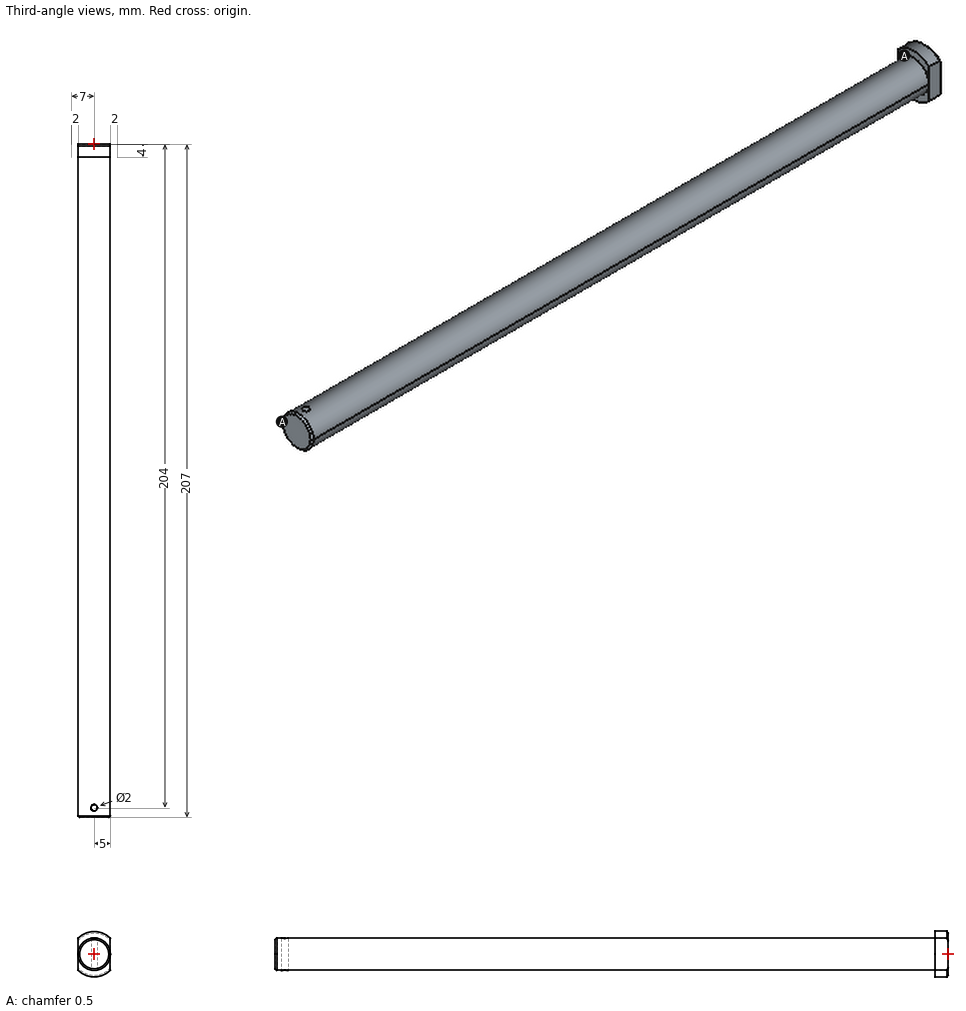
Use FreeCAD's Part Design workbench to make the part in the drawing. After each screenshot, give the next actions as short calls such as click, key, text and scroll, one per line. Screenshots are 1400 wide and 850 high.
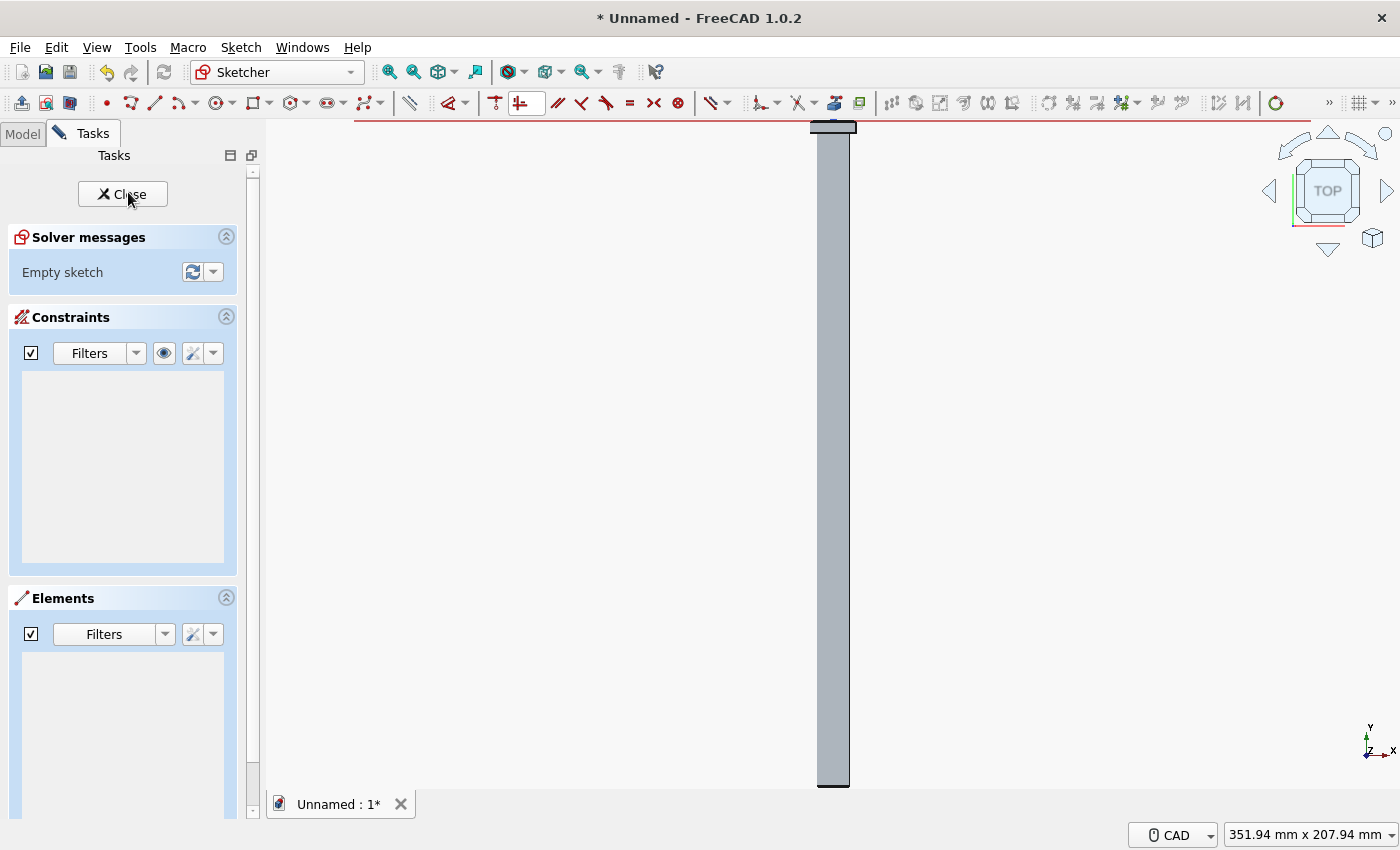
click(70, 104)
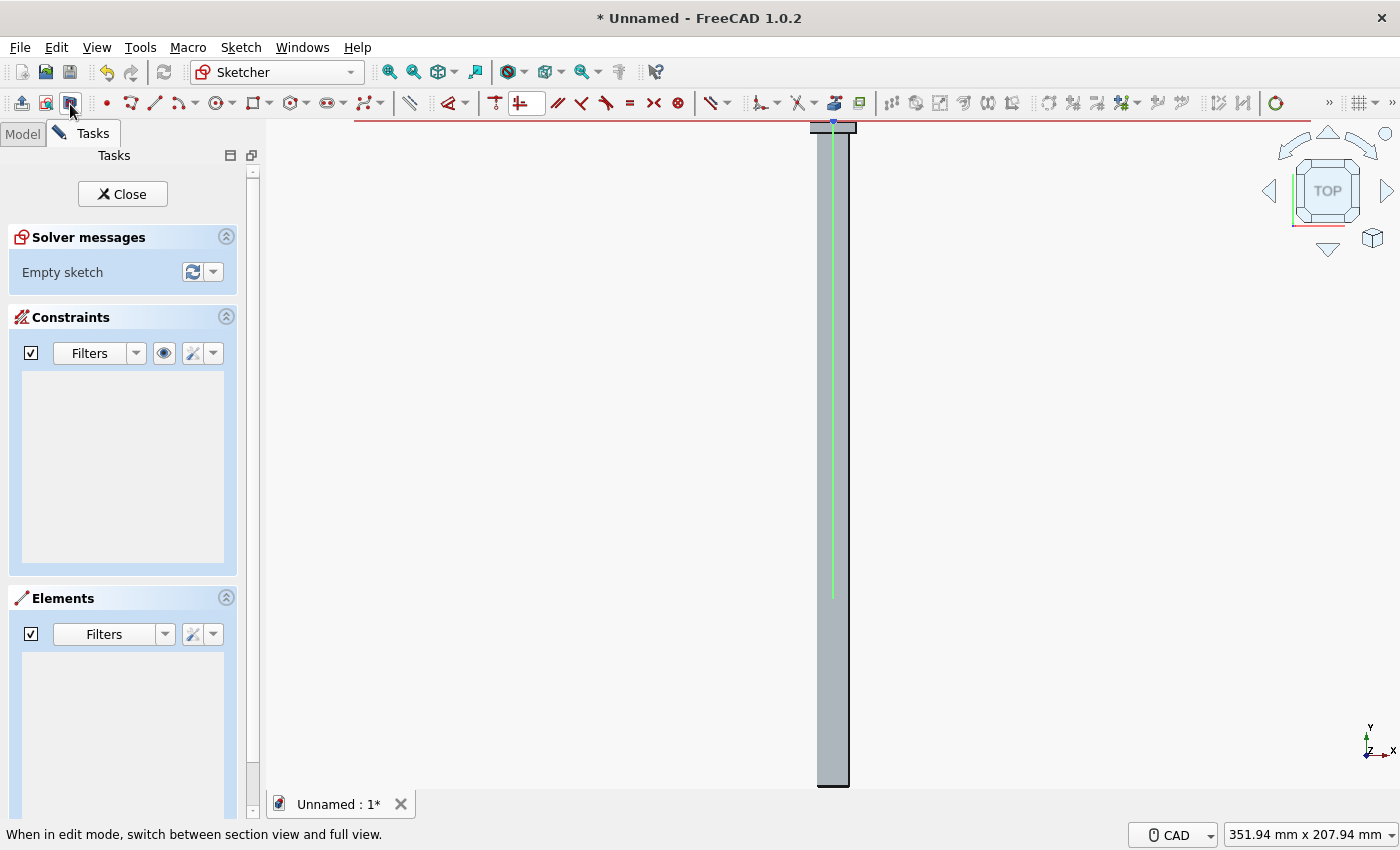
scroll(764, 454, down, 5)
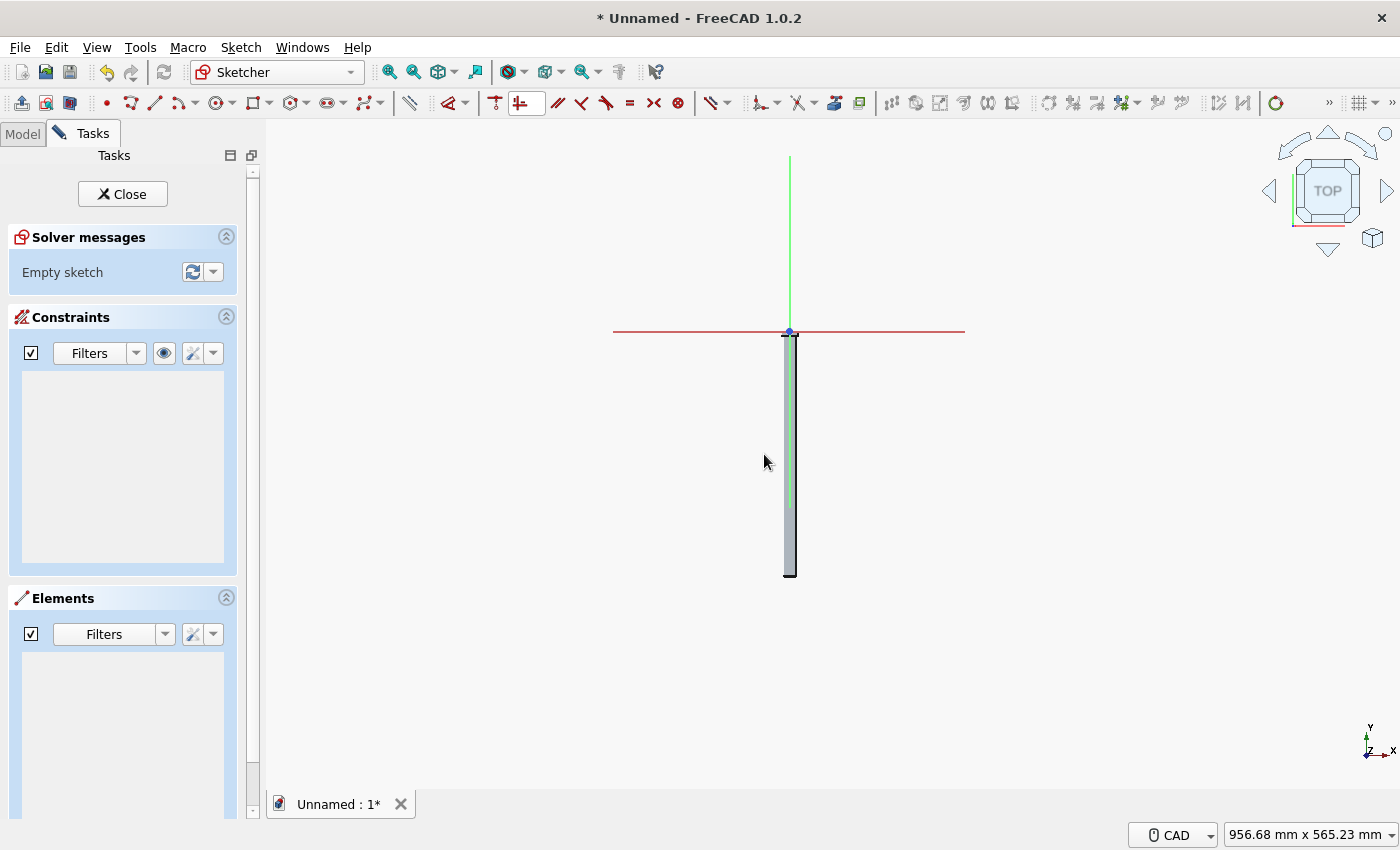
scroll(791, 580, up, 15)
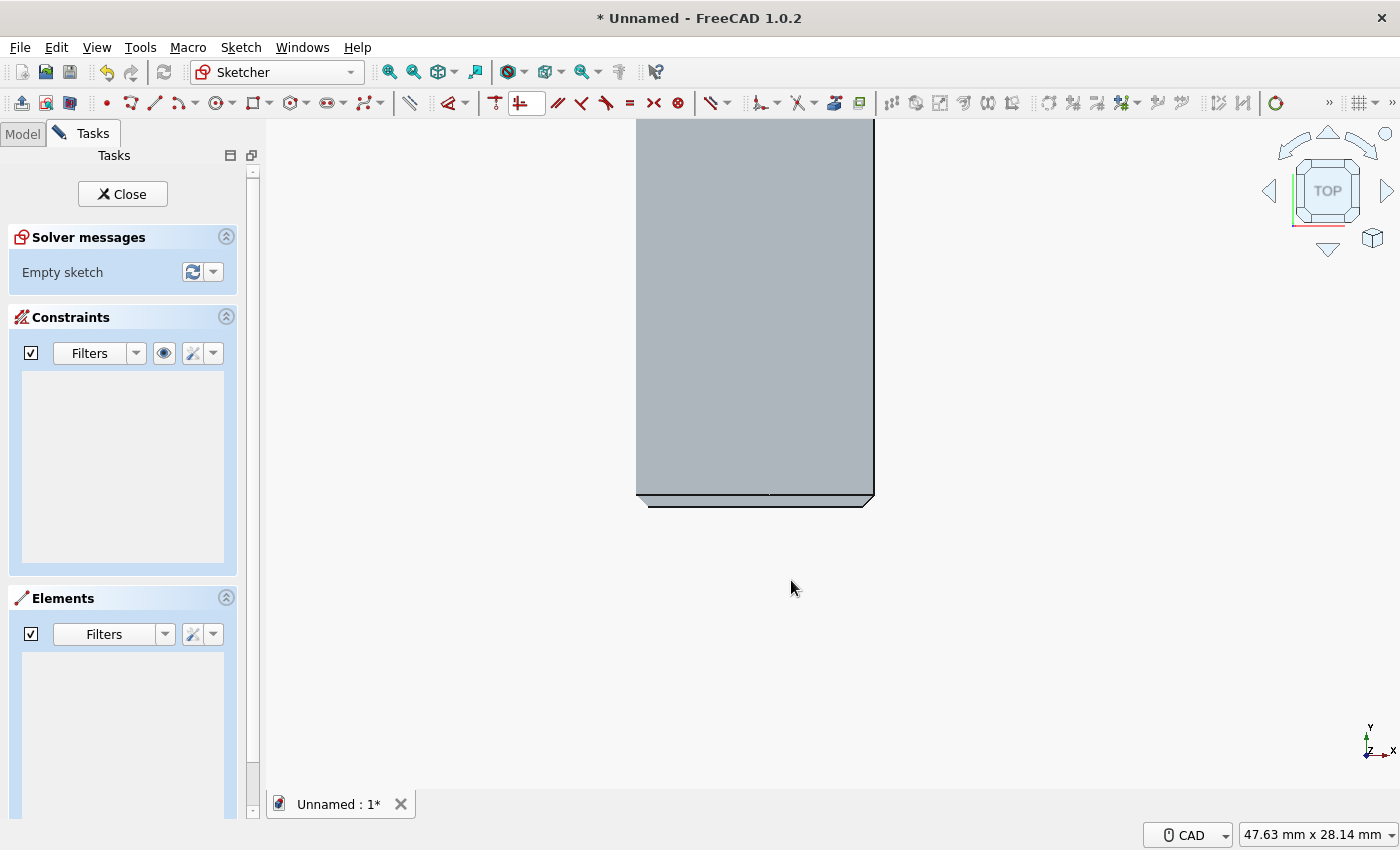
scroll(754, 433, up, 11)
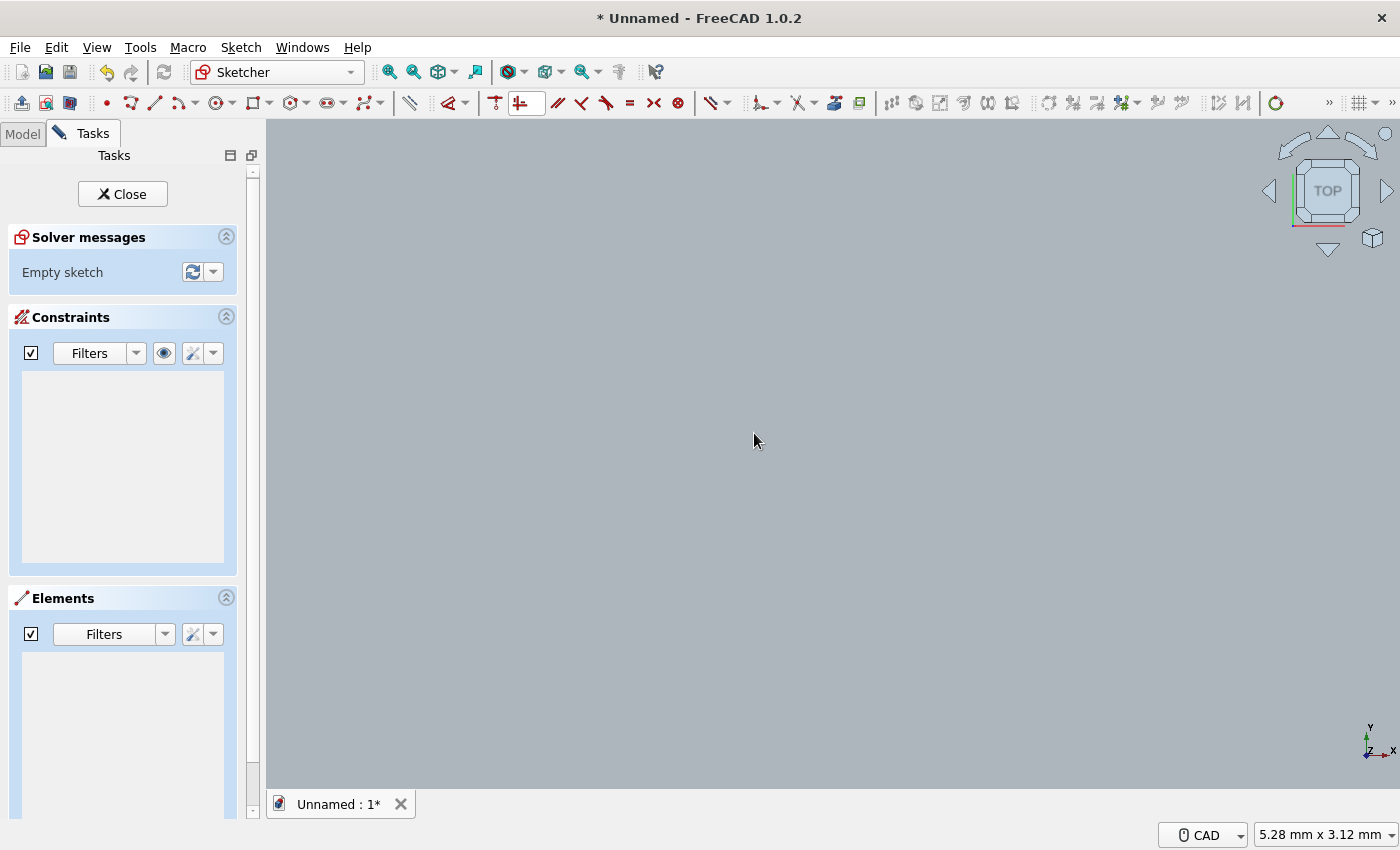
click(216, 104)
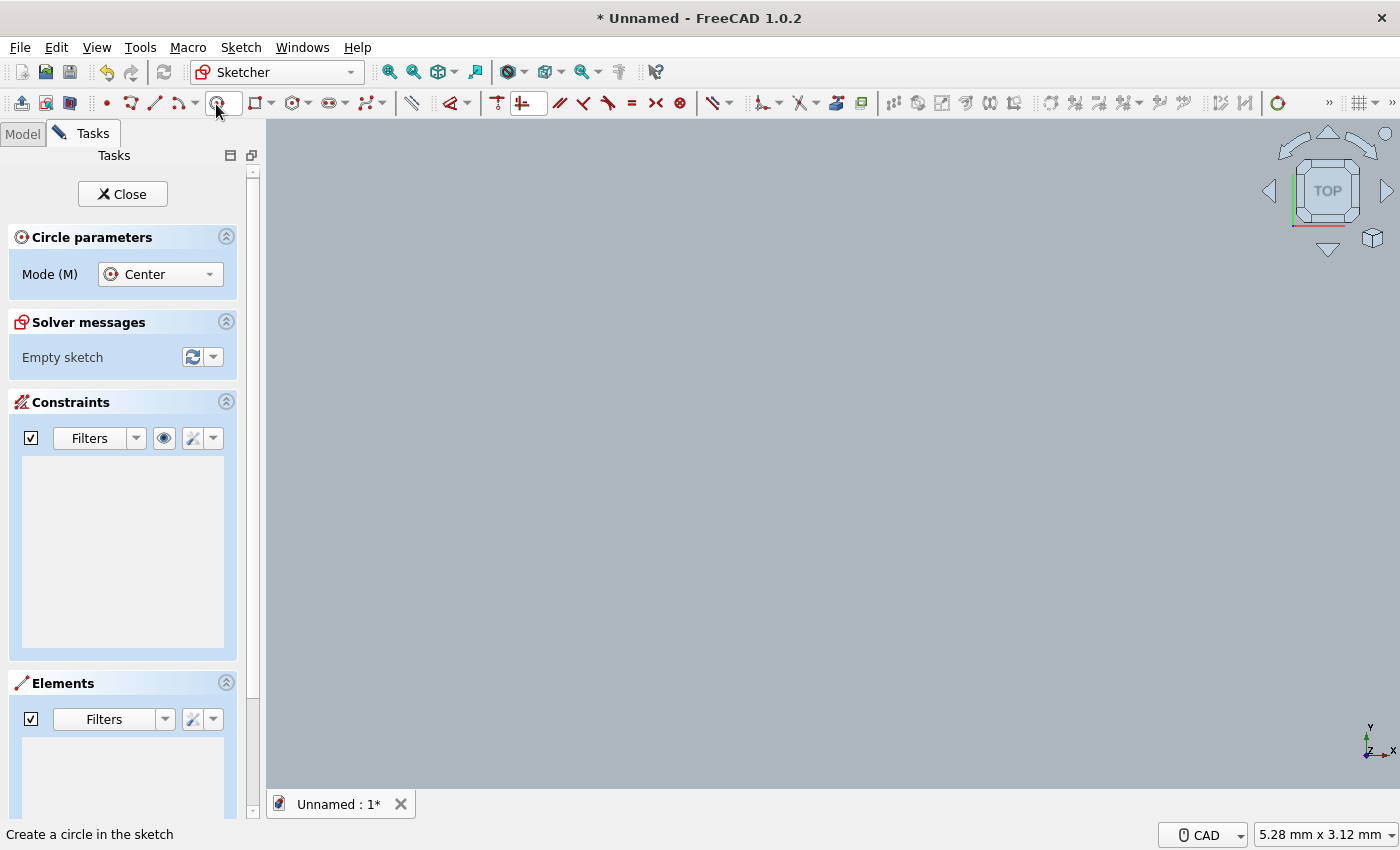
click(762, 449)
click(914, 297)
key(Escape)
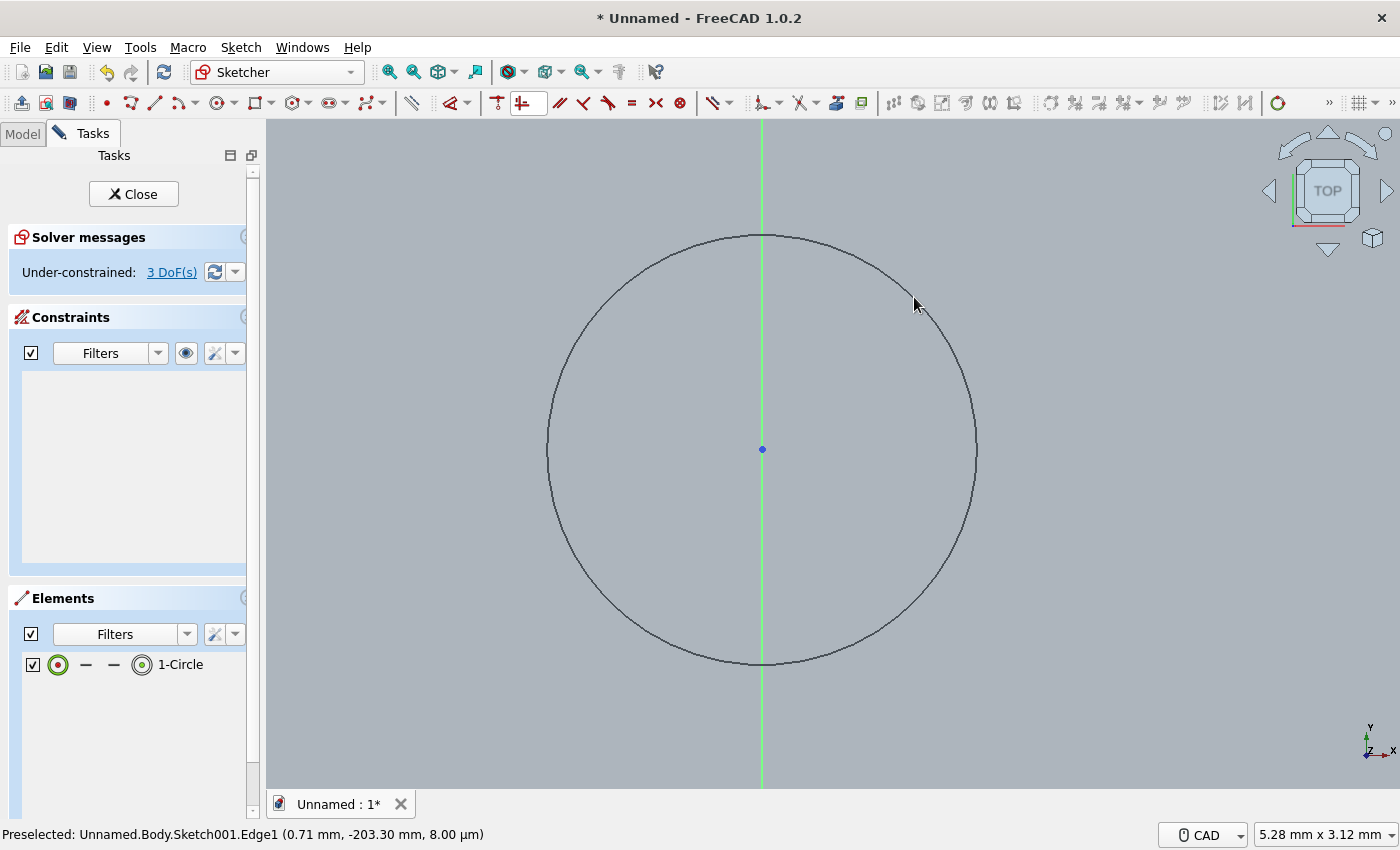
click(762, 450)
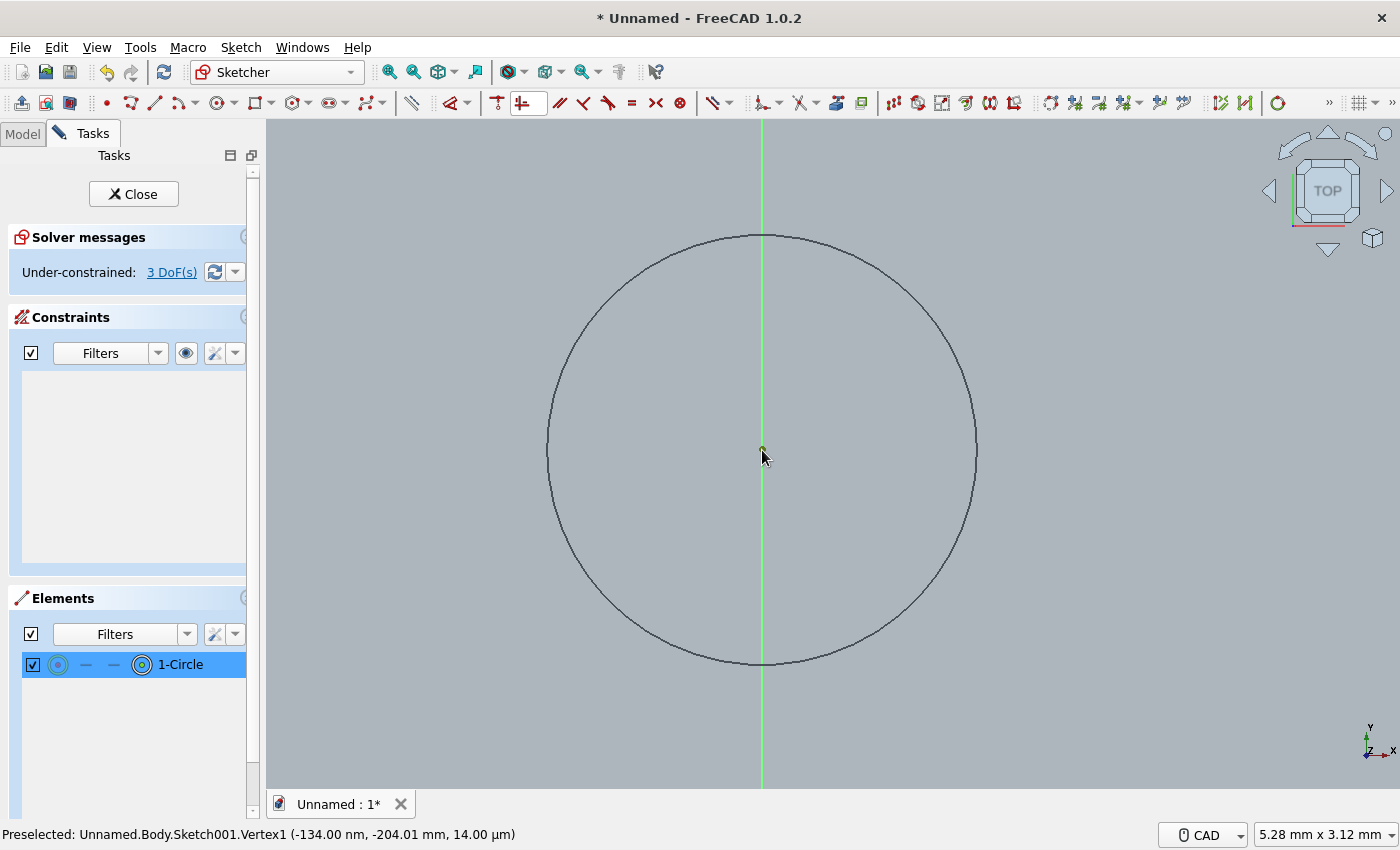
click(762, 717)